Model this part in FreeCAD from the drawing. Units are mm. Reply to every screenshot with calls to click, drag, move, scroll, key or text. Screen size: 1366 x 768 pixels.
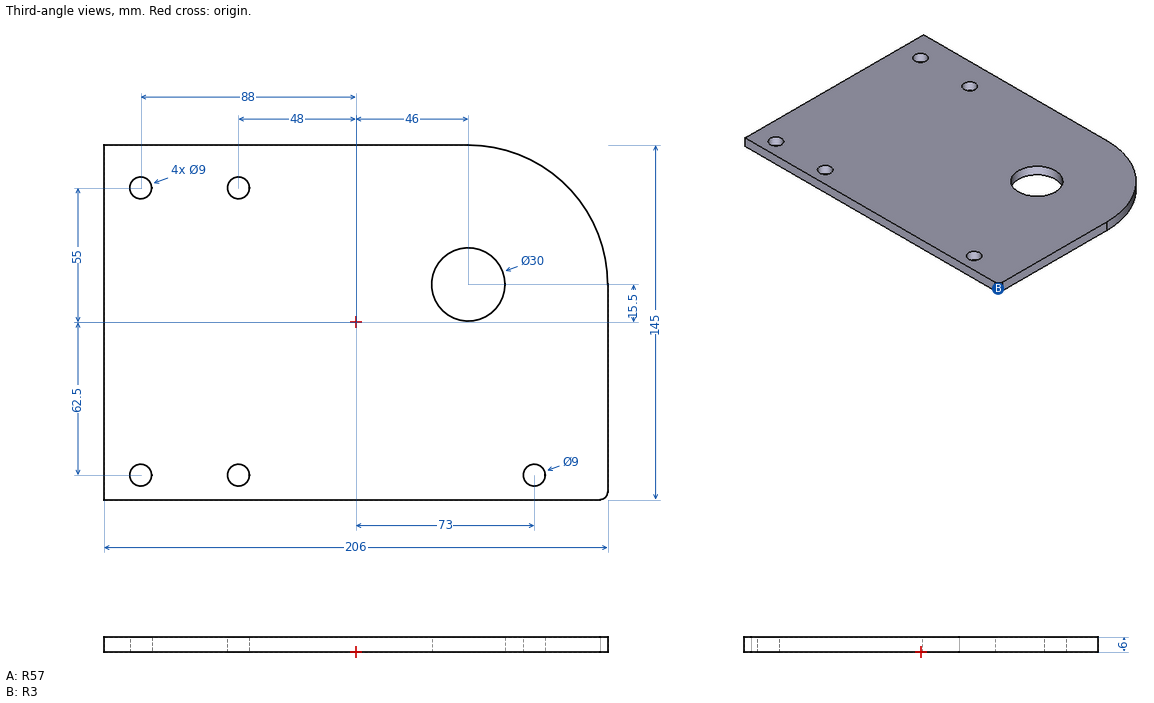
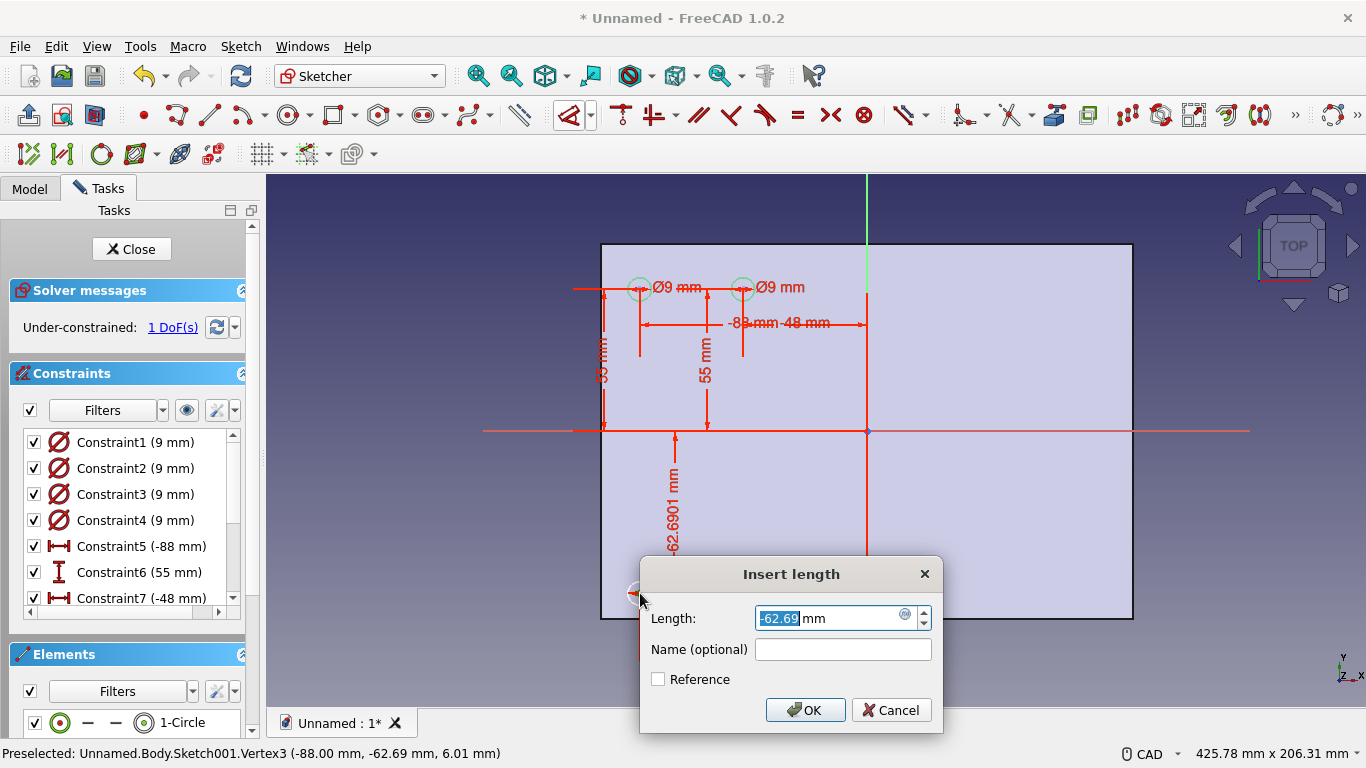
text(-62.5)
key(Return)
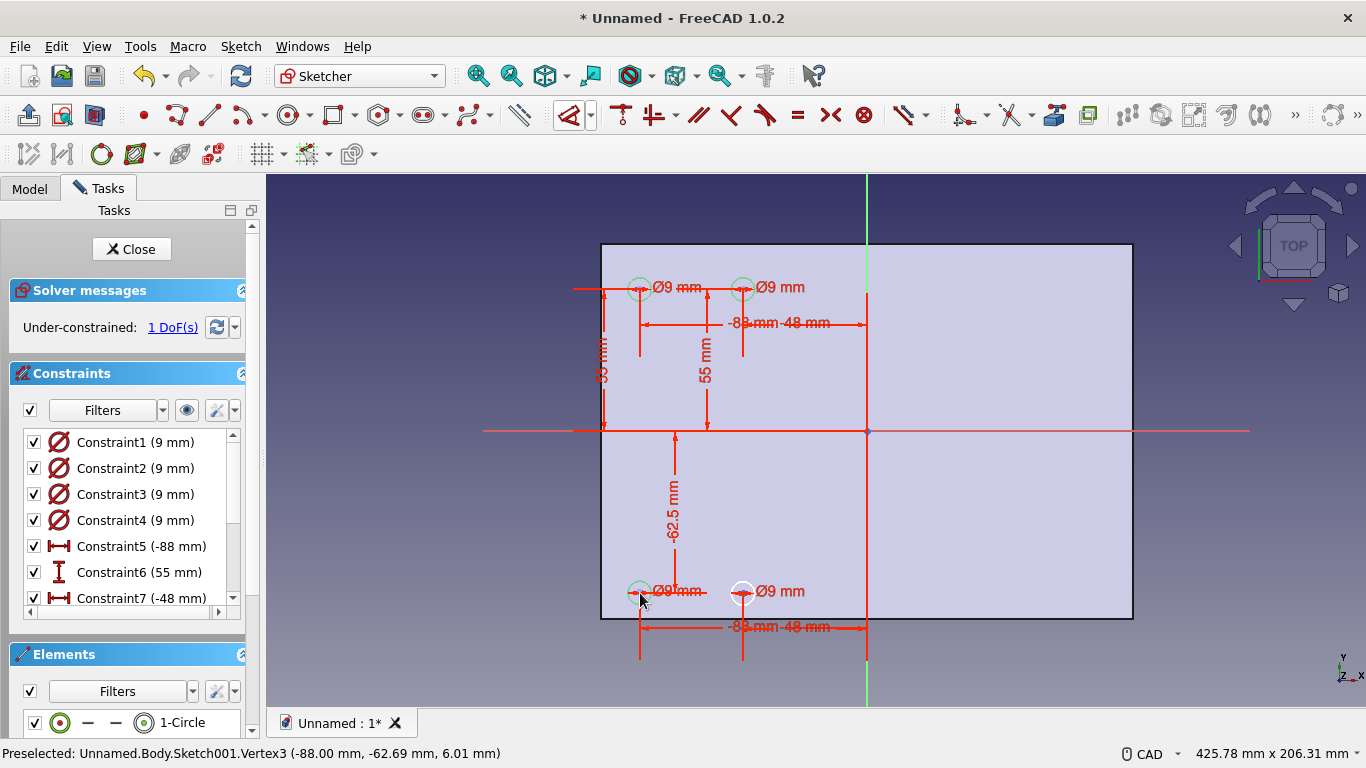
click(743, 593)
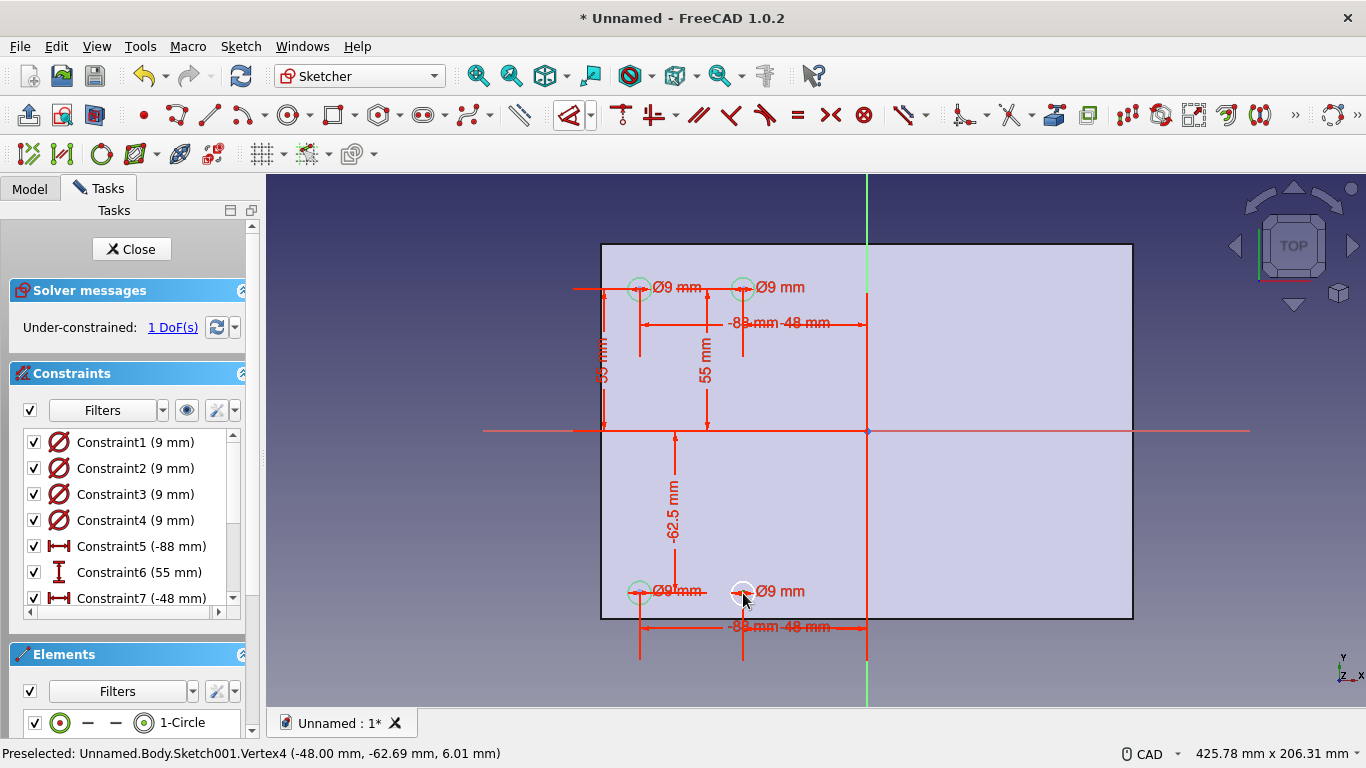
key(i)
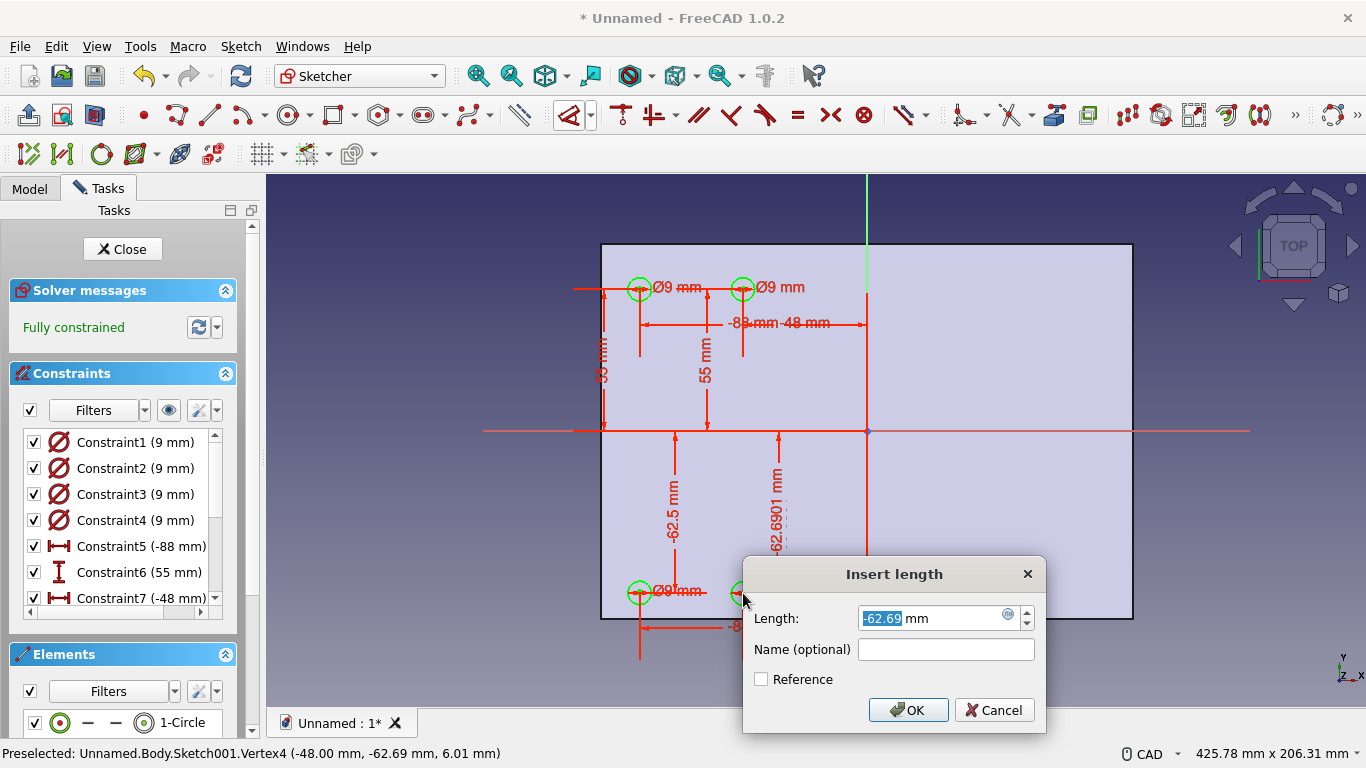
text(-62.5)
key(Return)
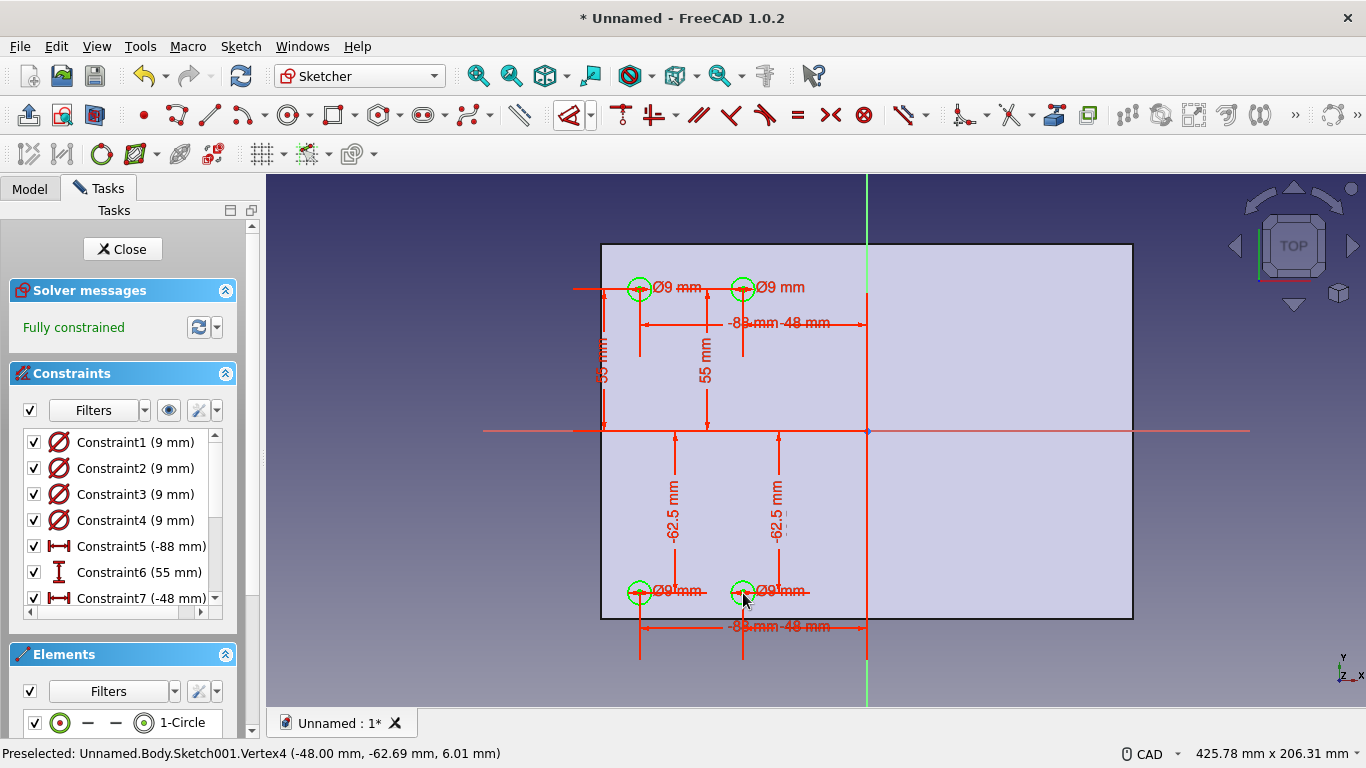
click(123, 249)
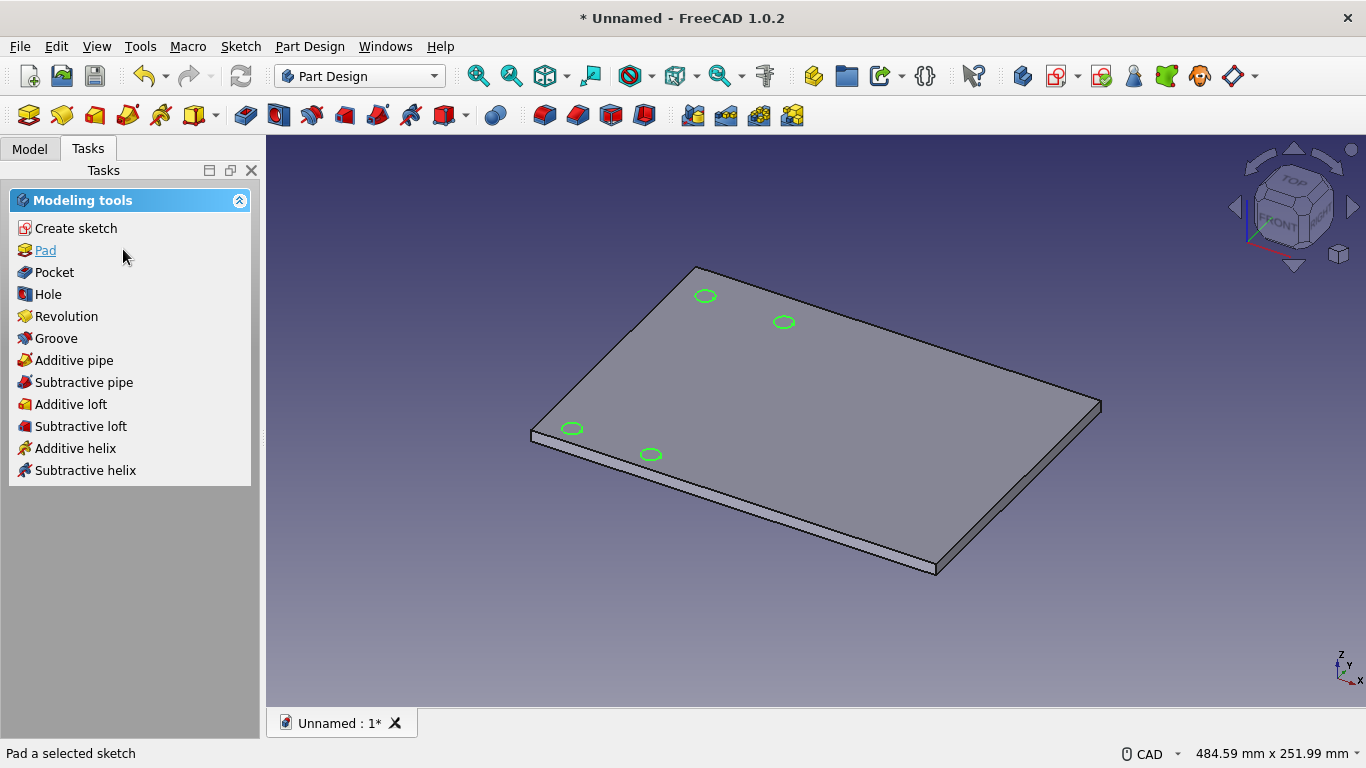
click(246, 116)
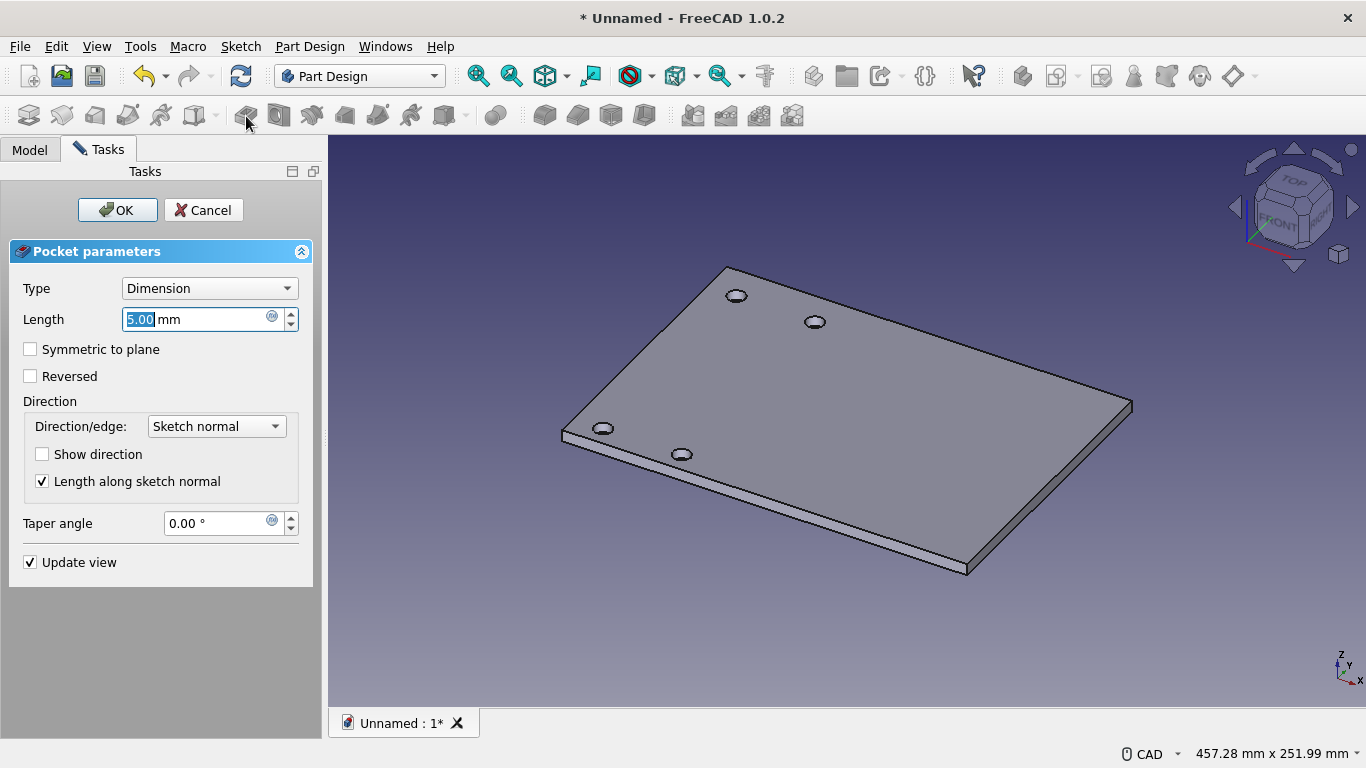
click(210, 288)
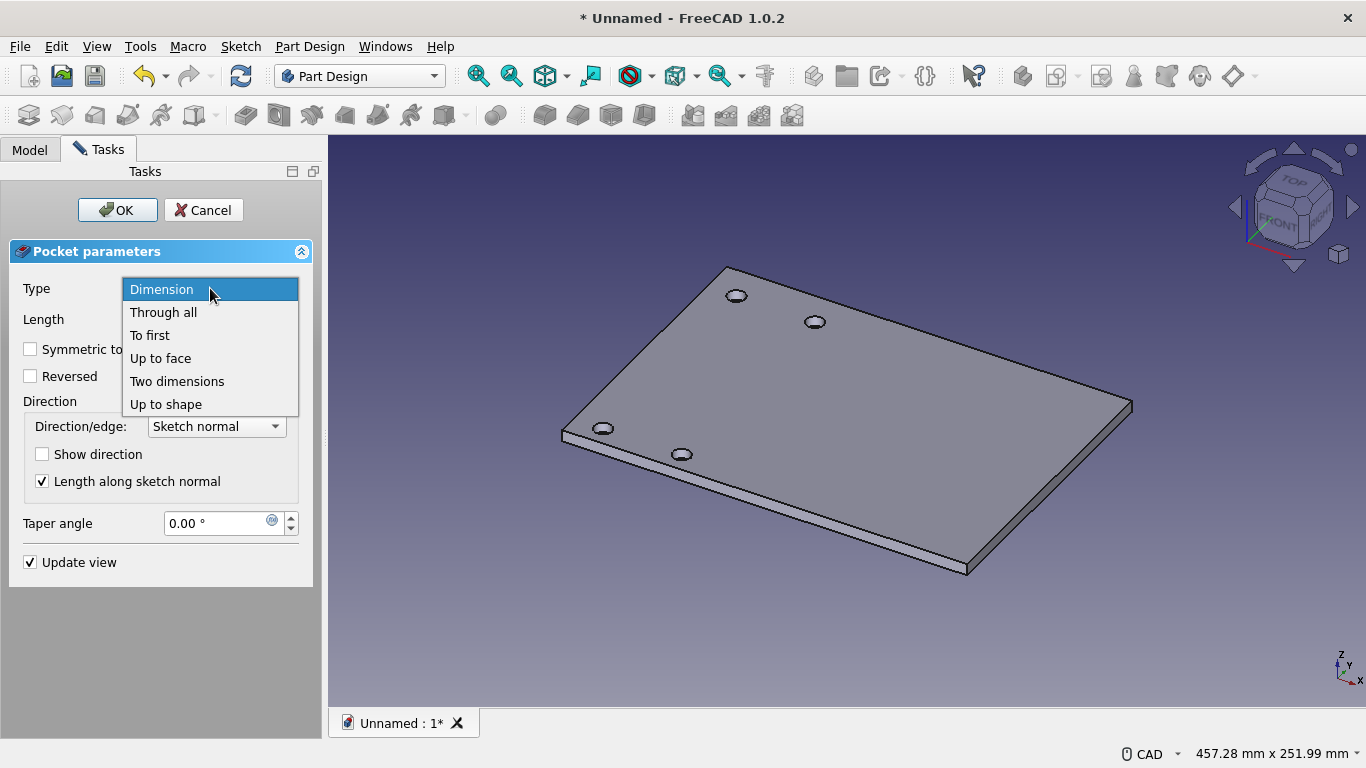
click(208, 312)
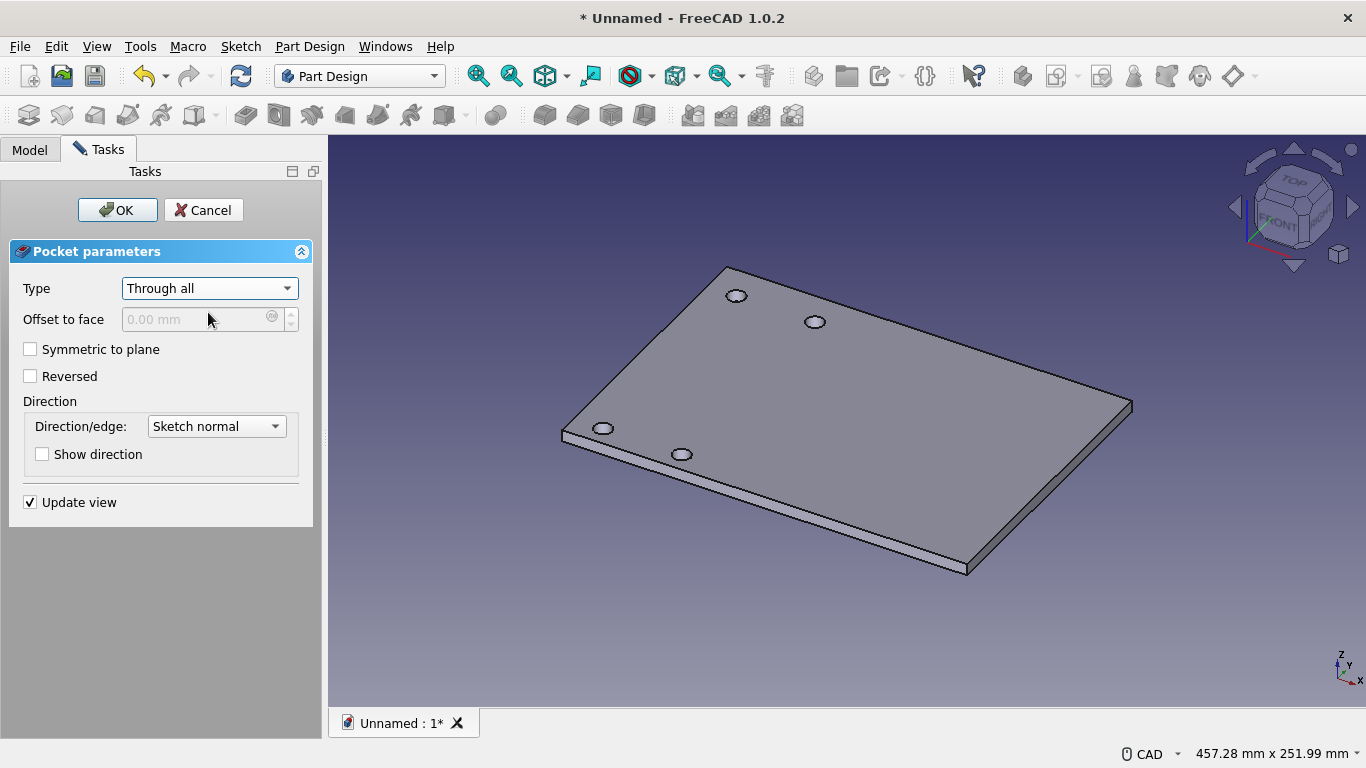
click(118, 210)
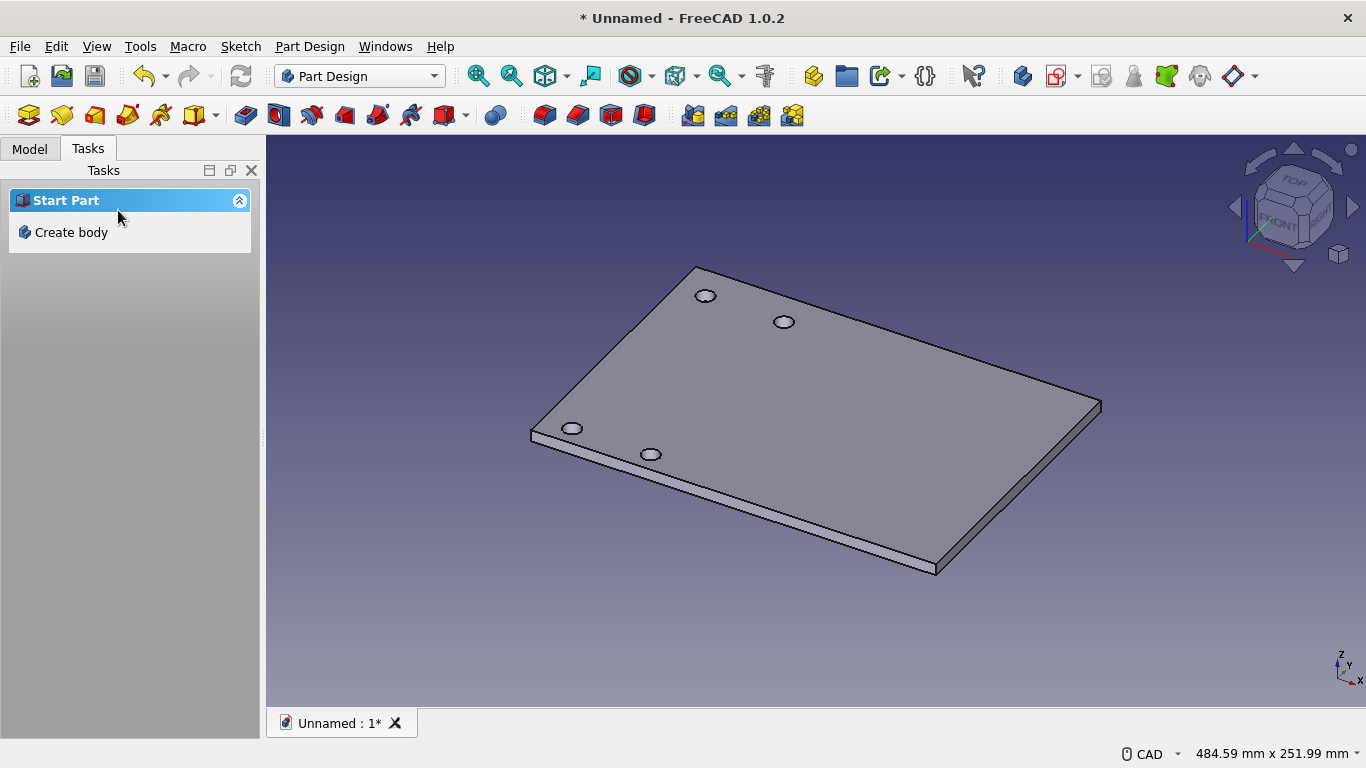
click(874, 434)